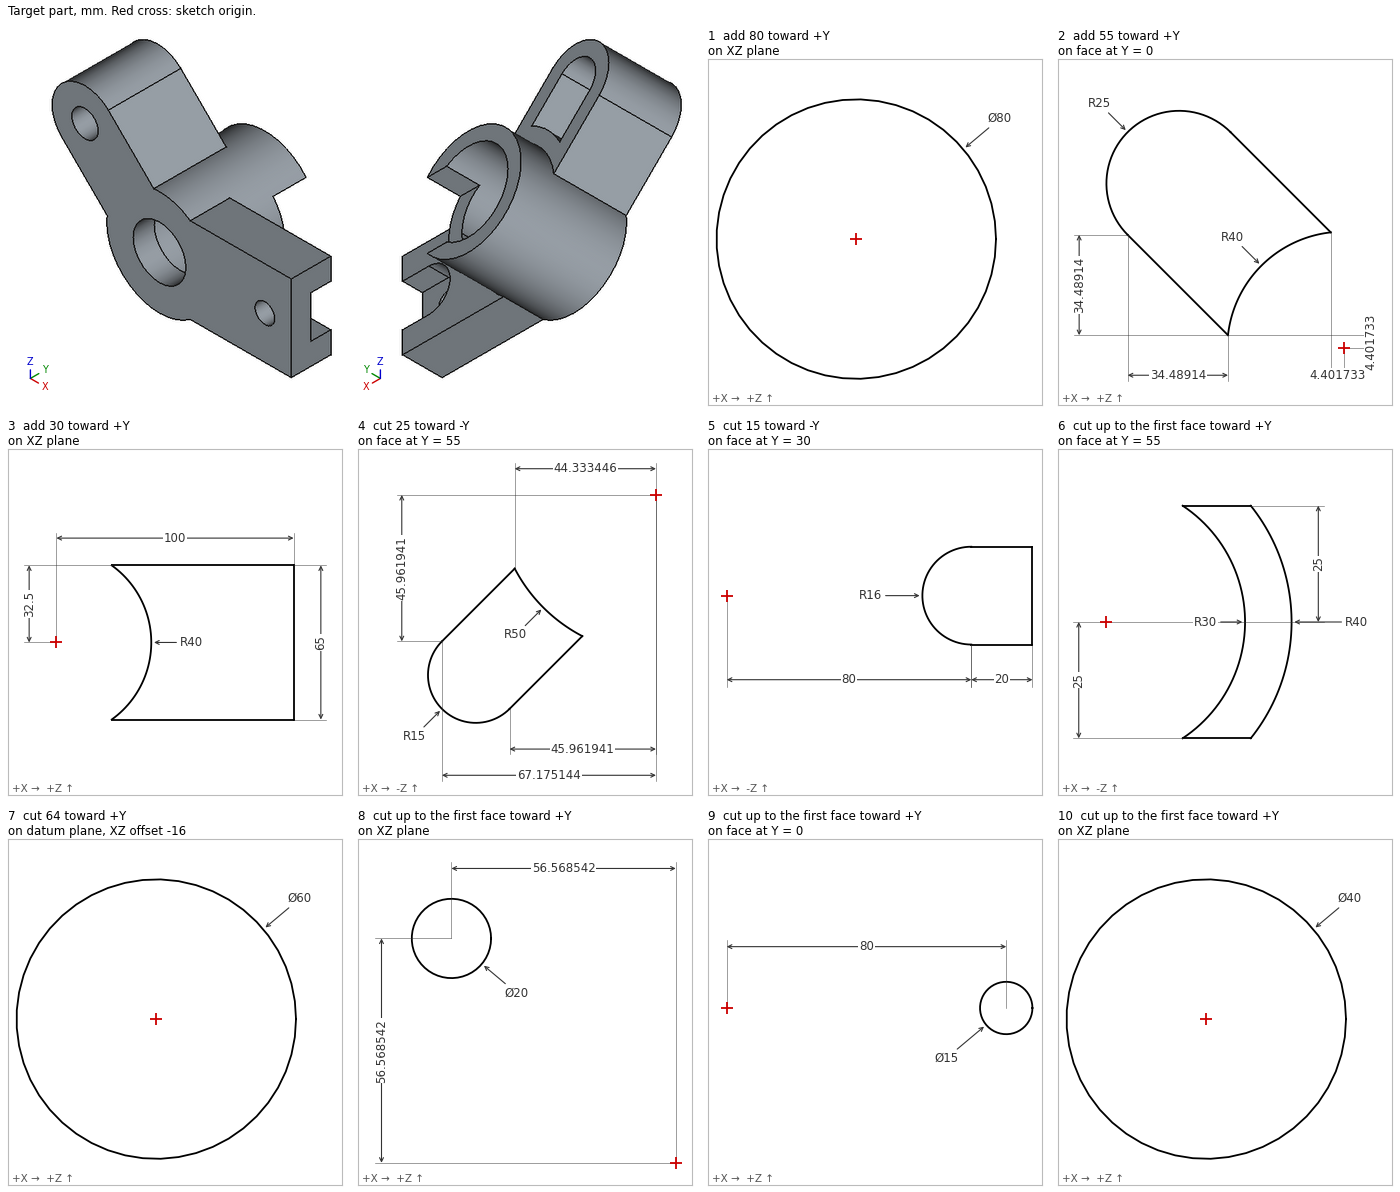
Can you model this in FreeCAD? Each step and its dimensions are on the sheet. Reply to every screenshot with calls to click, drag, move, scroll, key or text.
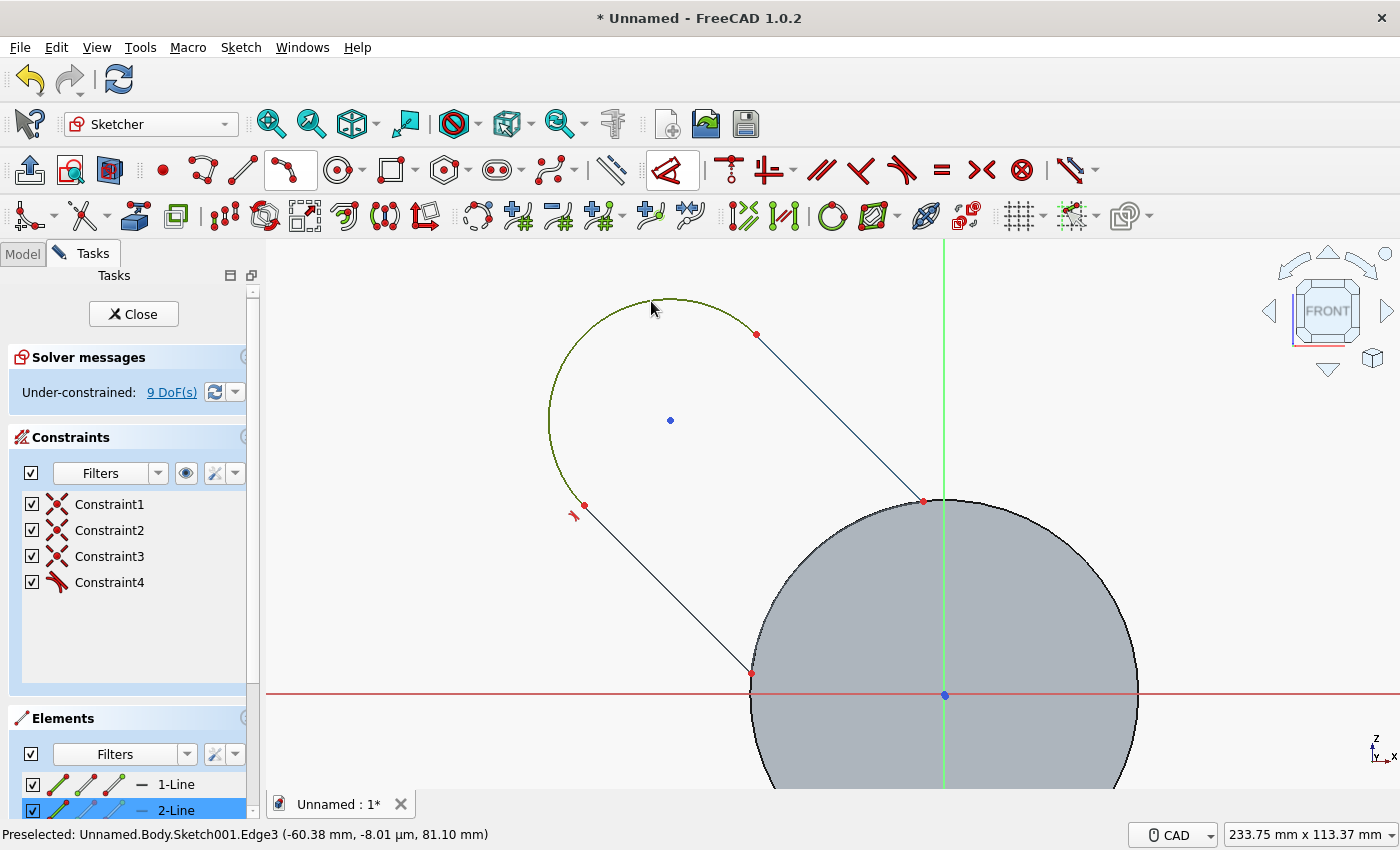
key(t)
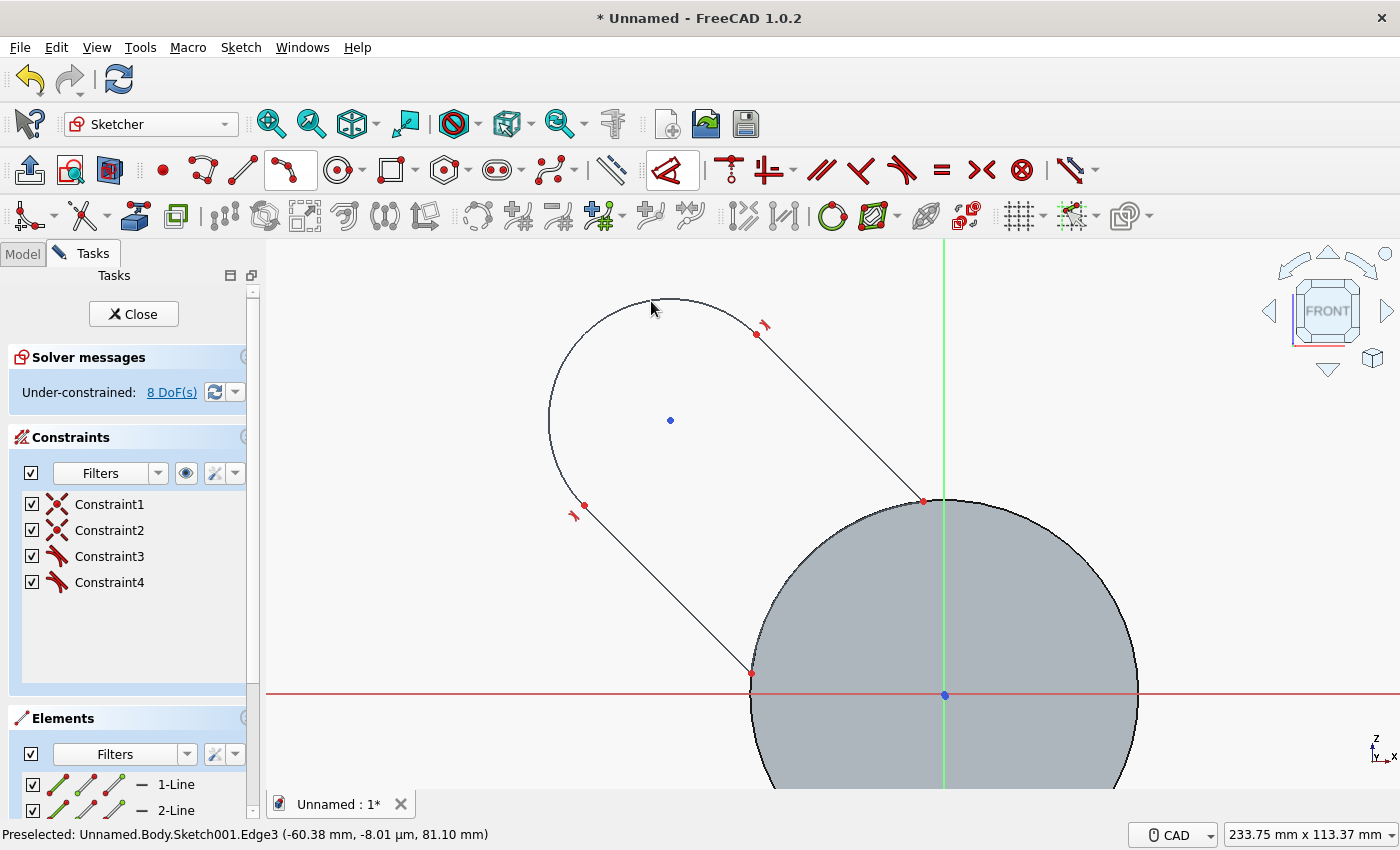
drag(934, 684, 955, 706)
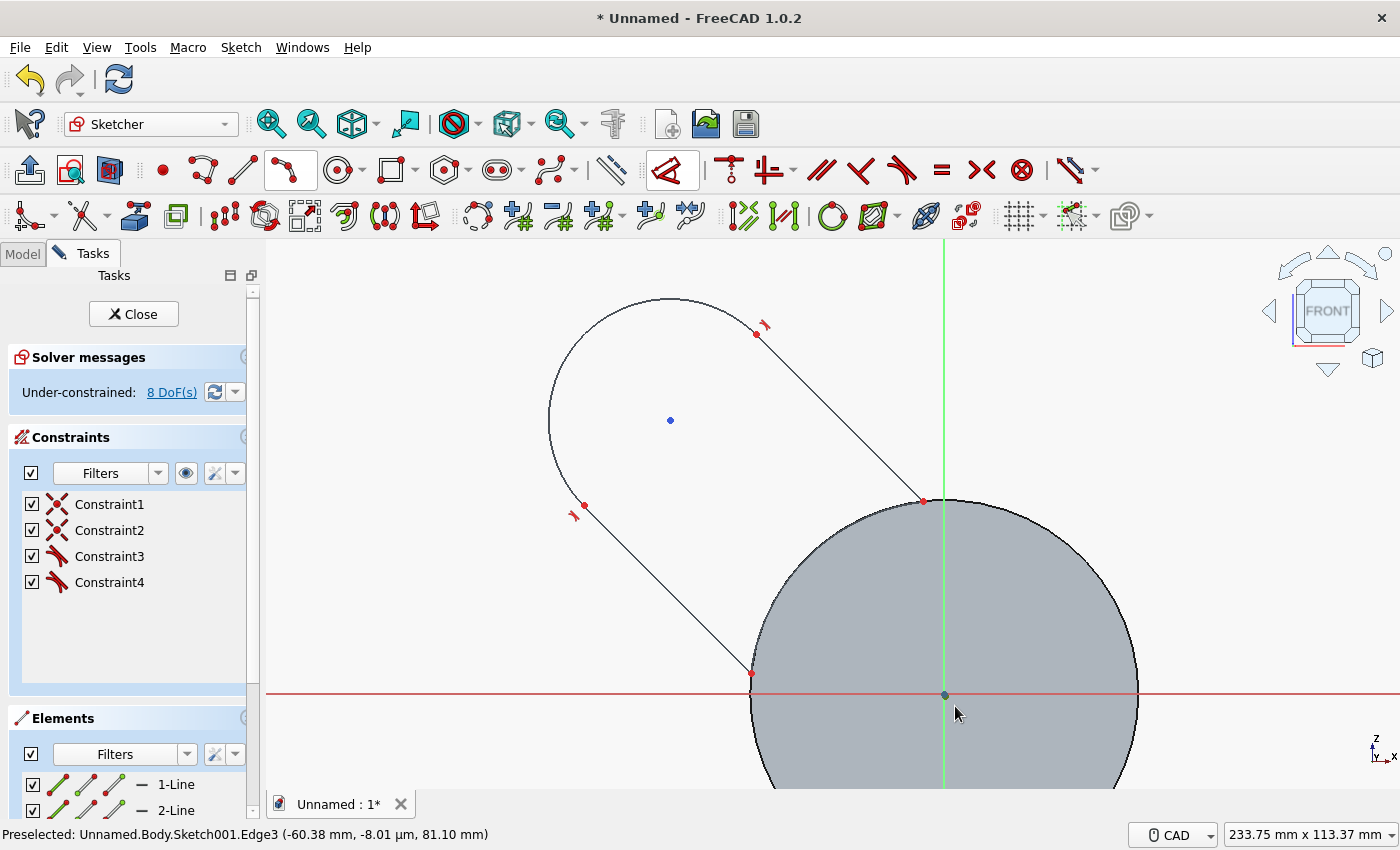
click(730, 170)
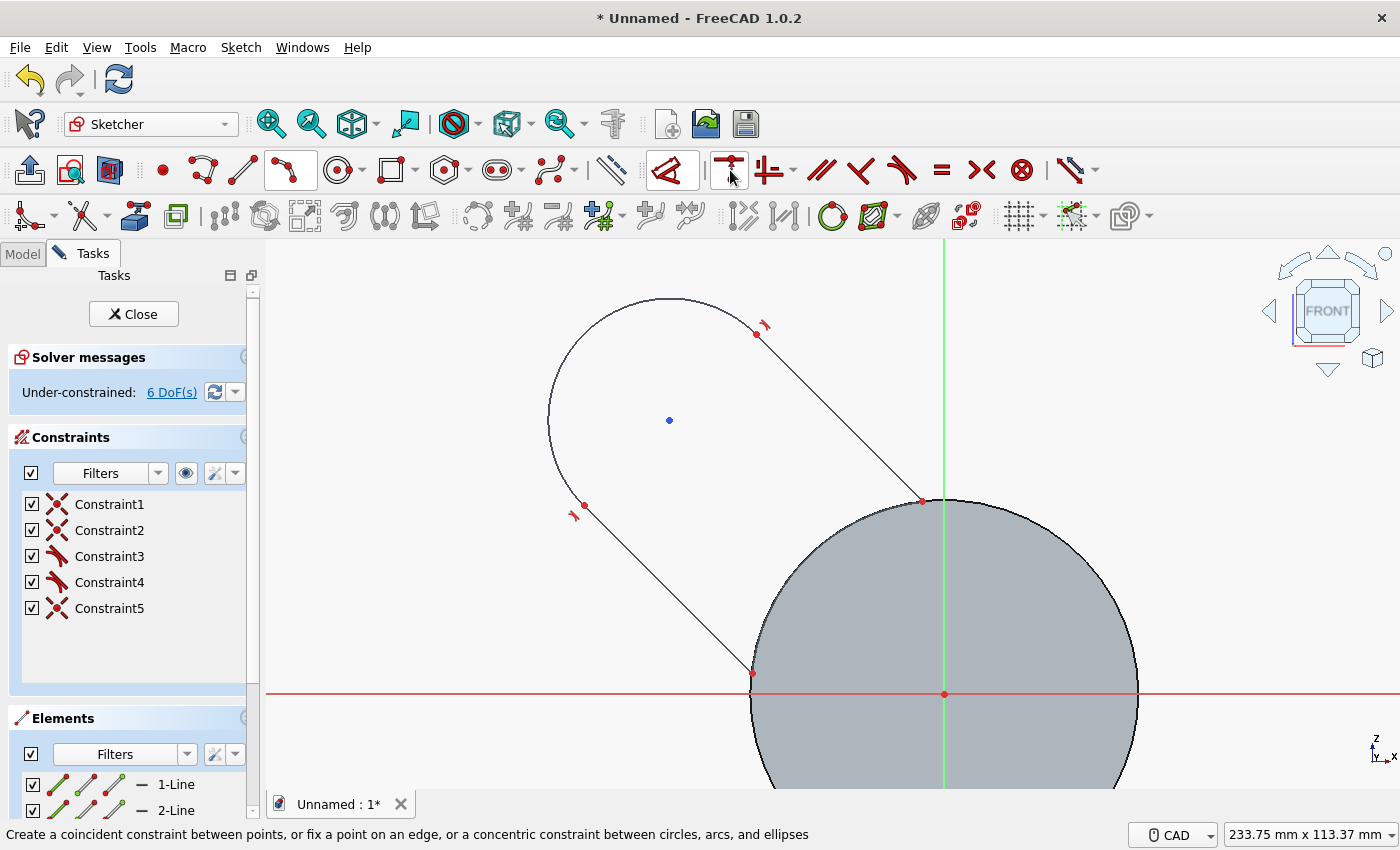
click(651, 300)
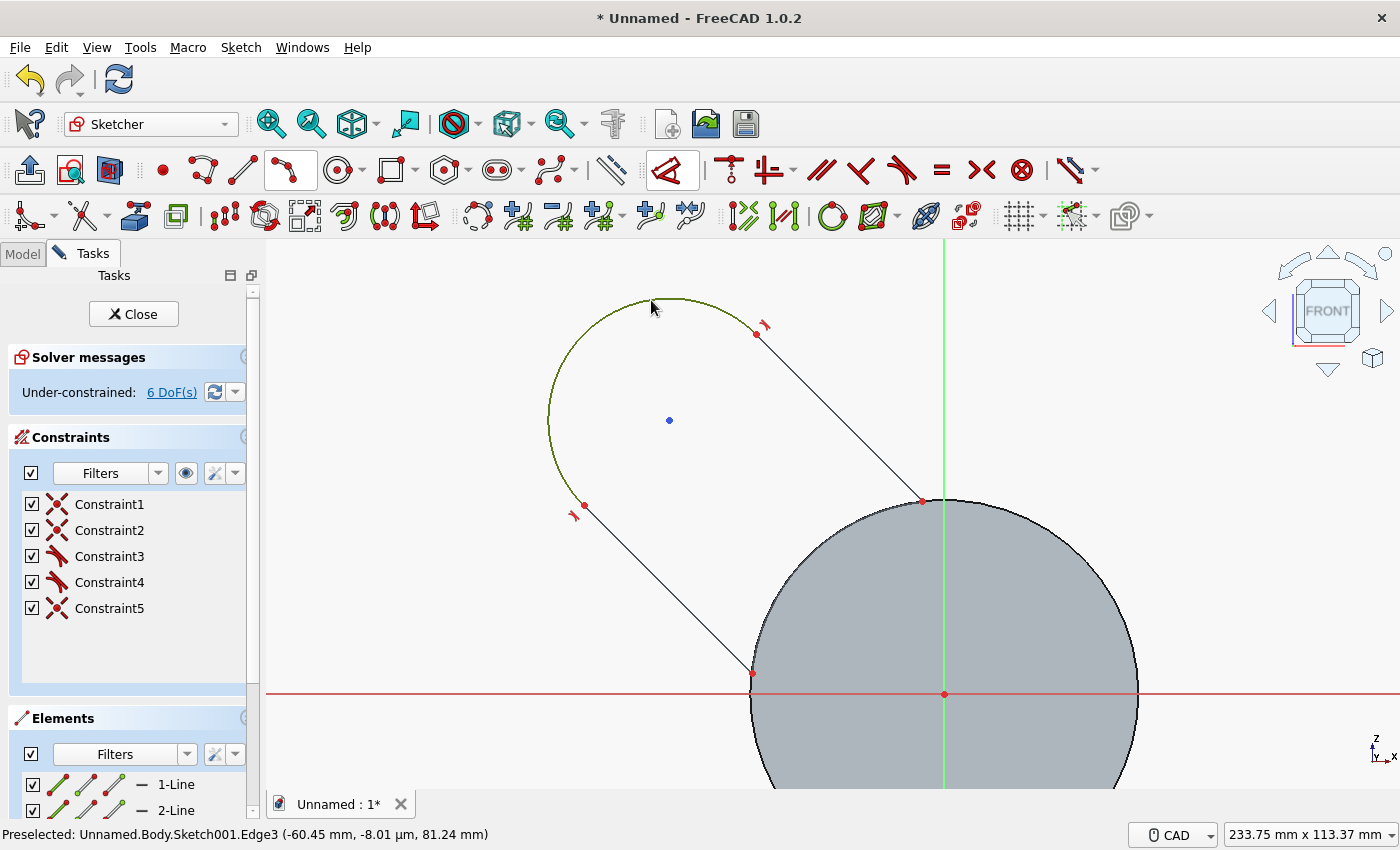
click(694, 170)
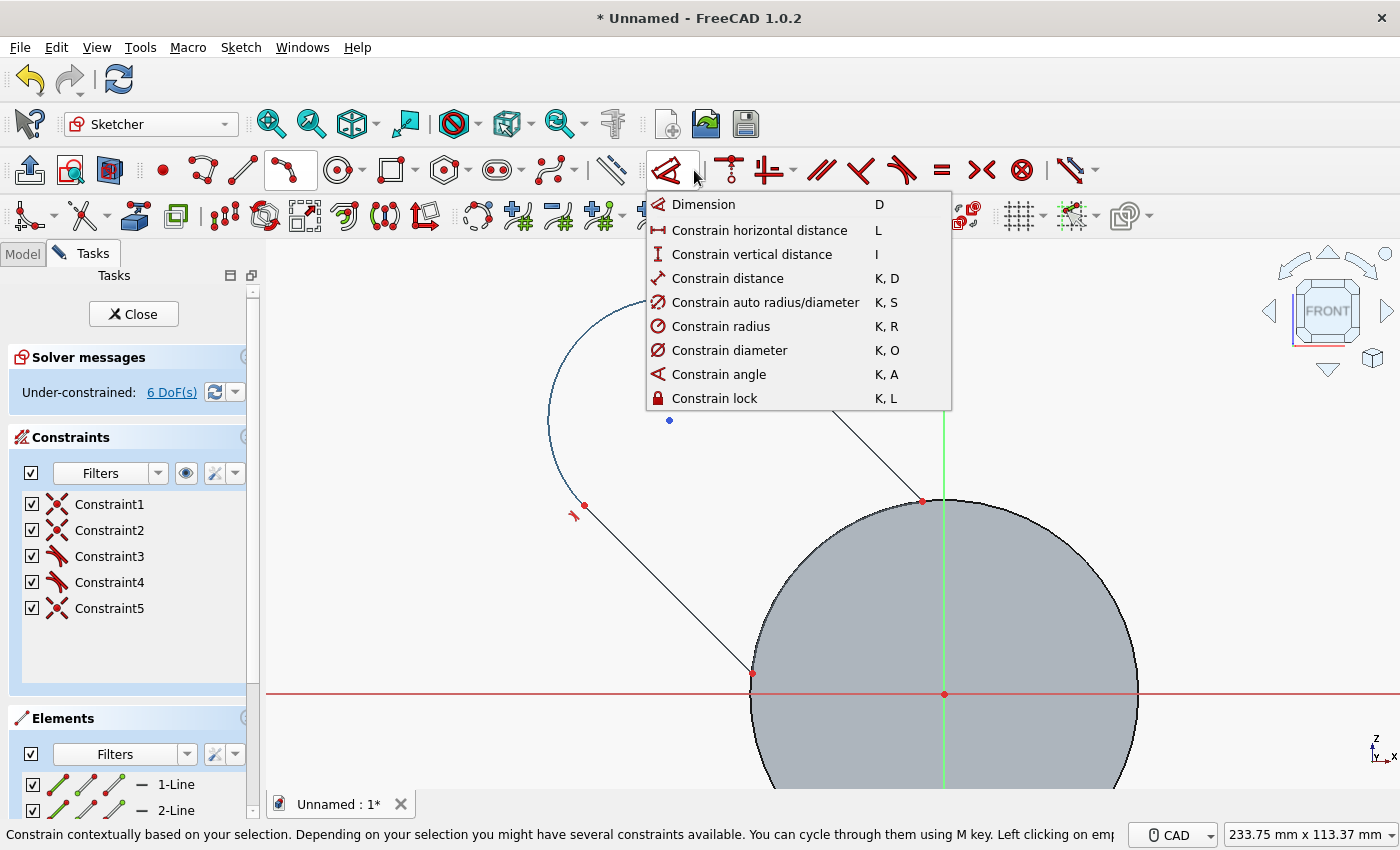
click(799, 326)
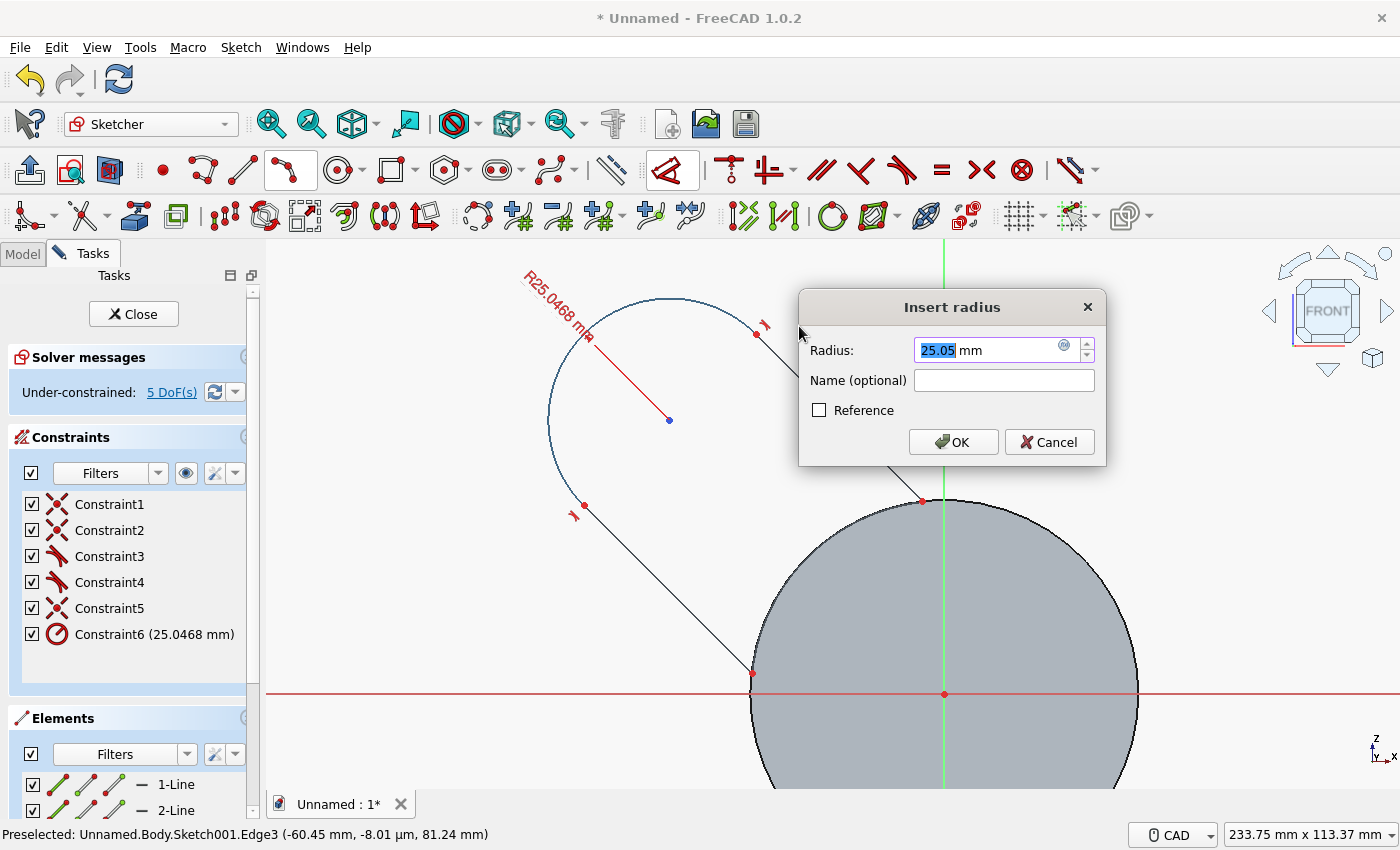
text(25)
key(Return)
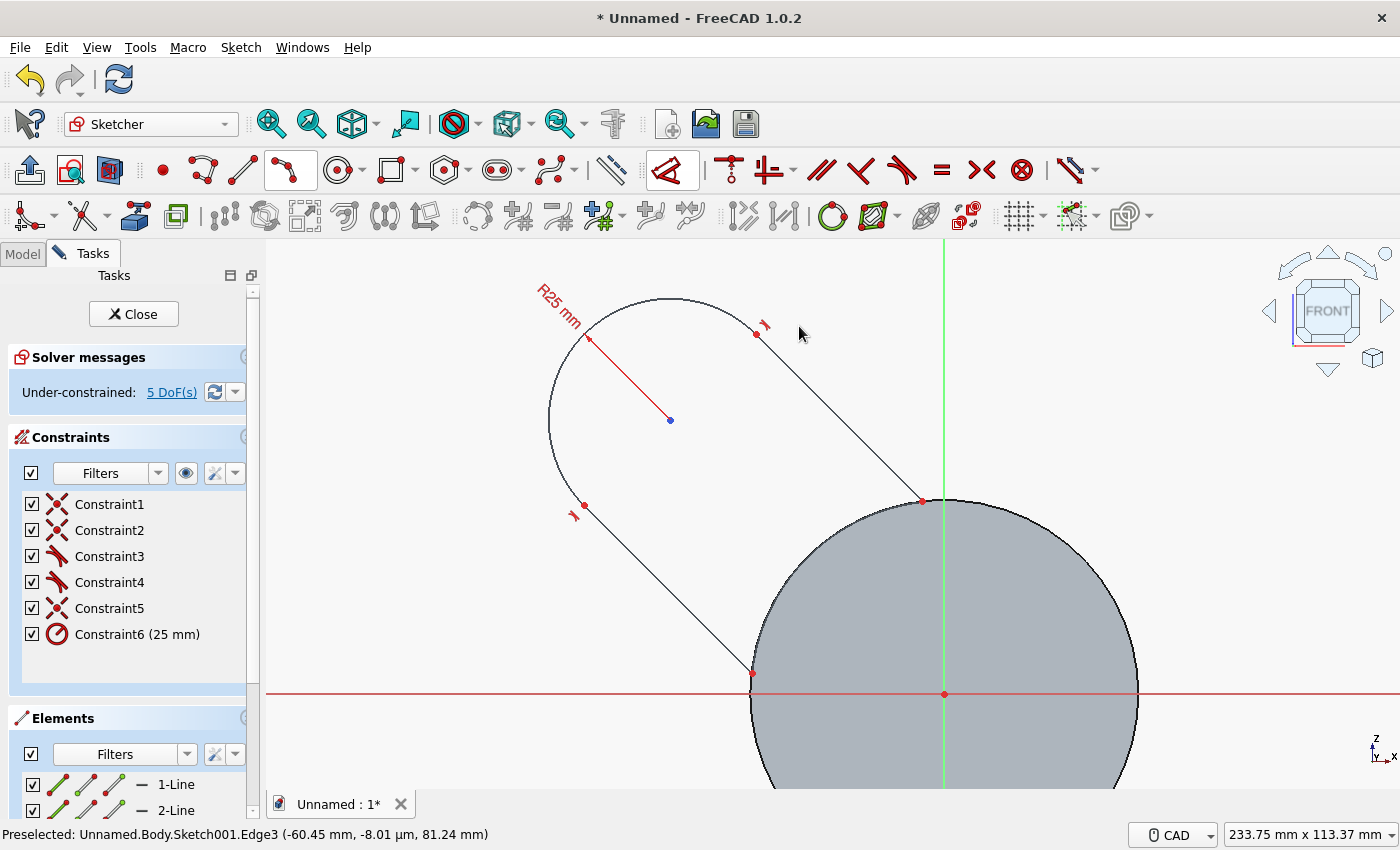
click(849, 526)